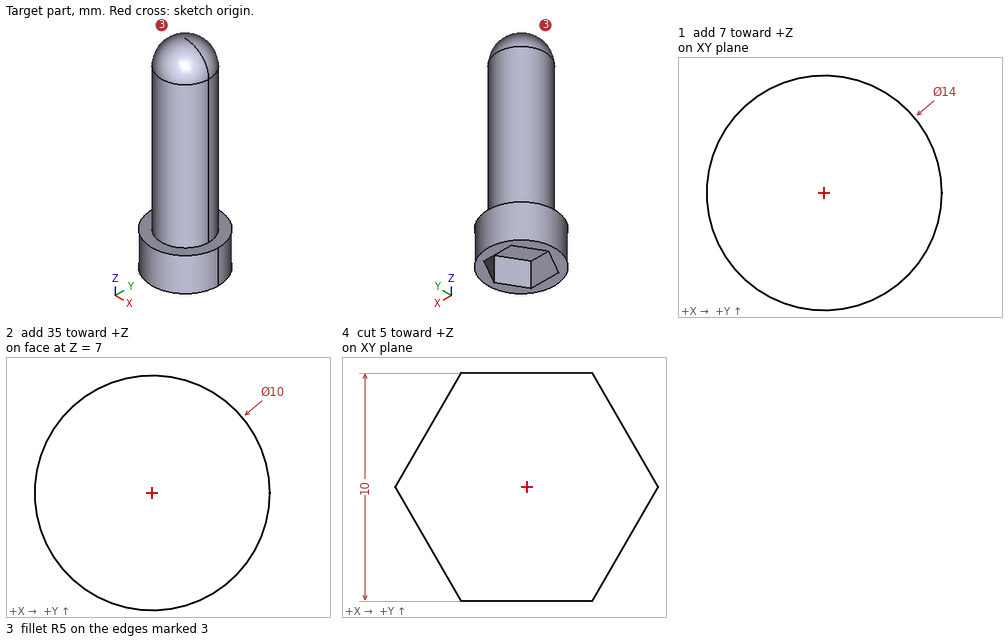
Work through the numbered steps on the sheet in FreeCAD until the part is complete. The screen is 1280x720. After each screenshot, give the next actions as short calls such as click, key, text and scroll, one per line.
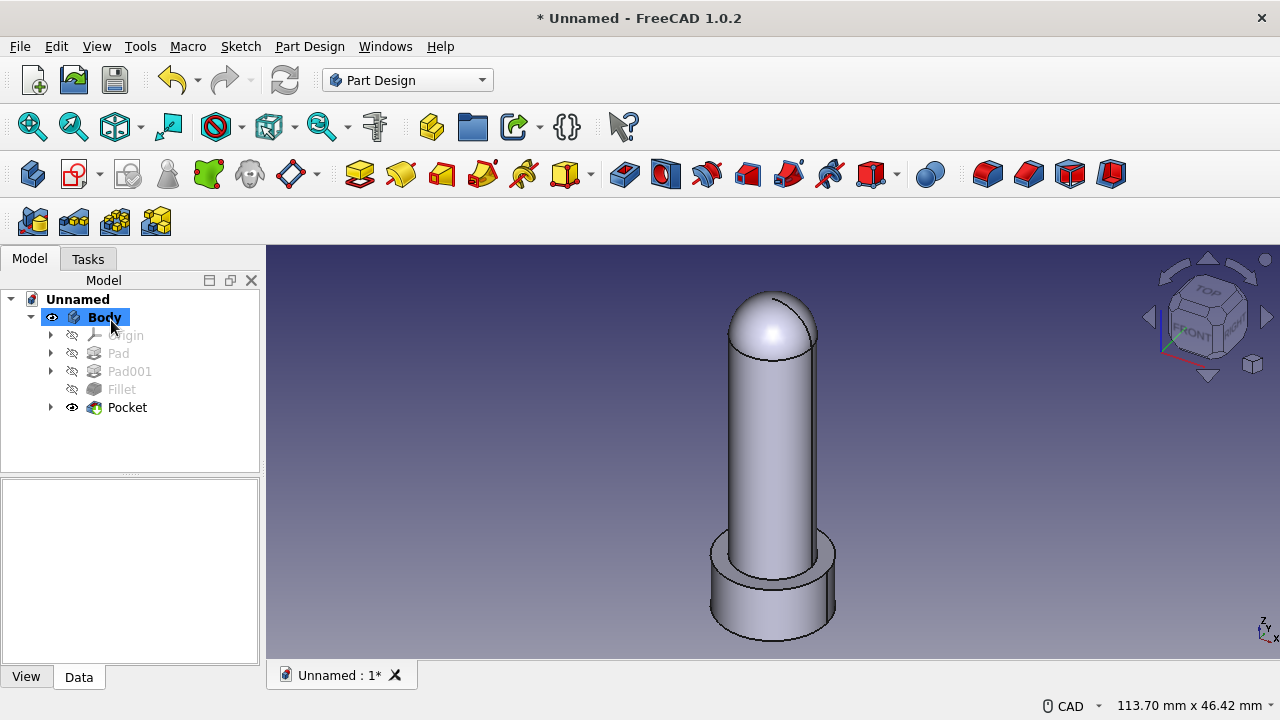
key(0)